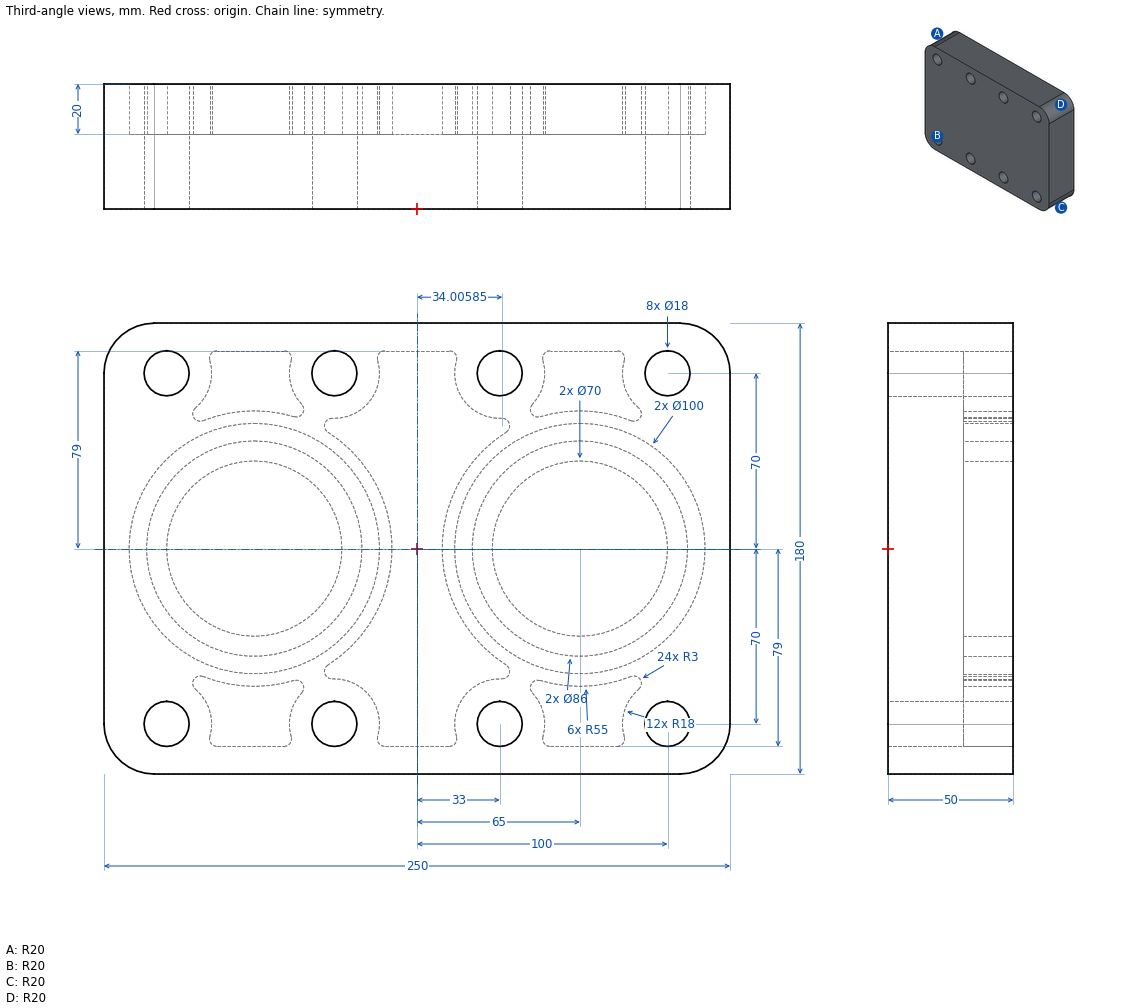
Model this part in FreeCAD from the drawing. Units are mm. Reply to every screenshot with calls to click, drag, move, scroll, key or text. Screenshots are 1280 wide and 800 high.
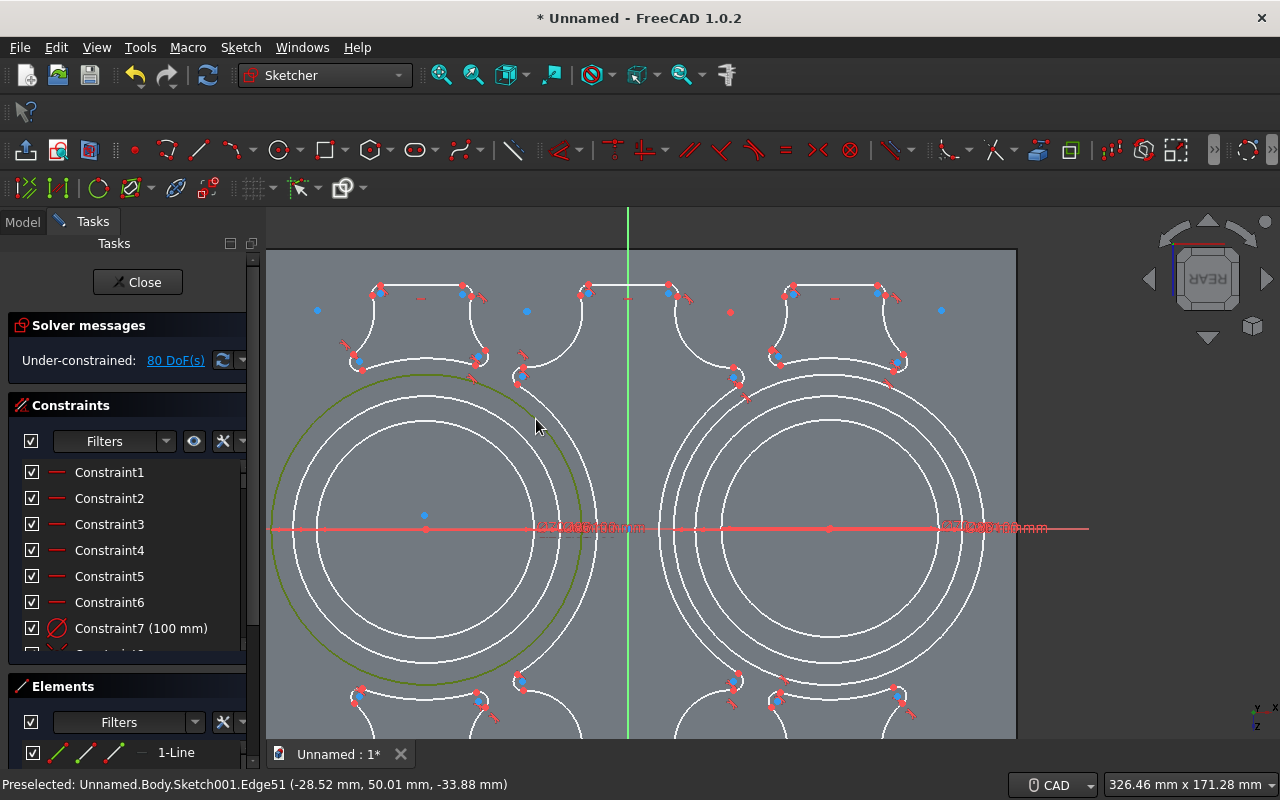
click(583, 596)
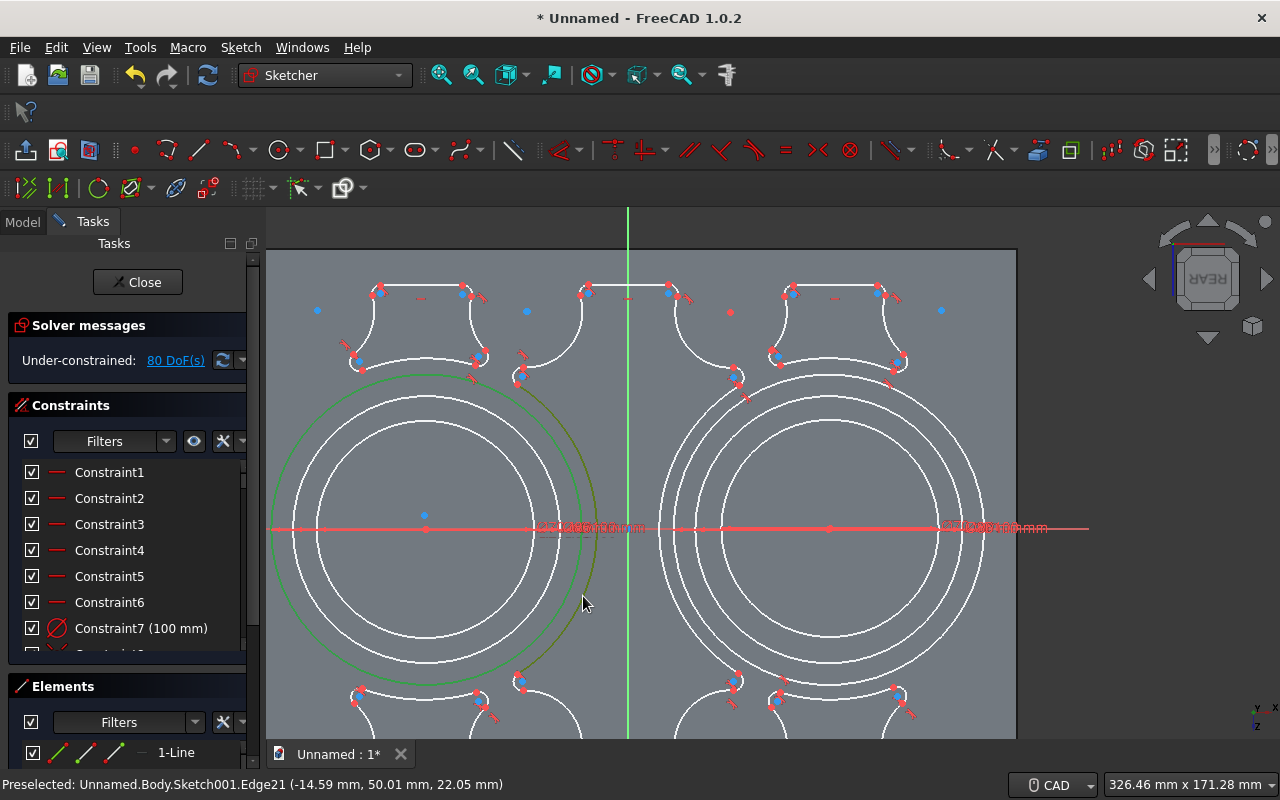
click(614, 150)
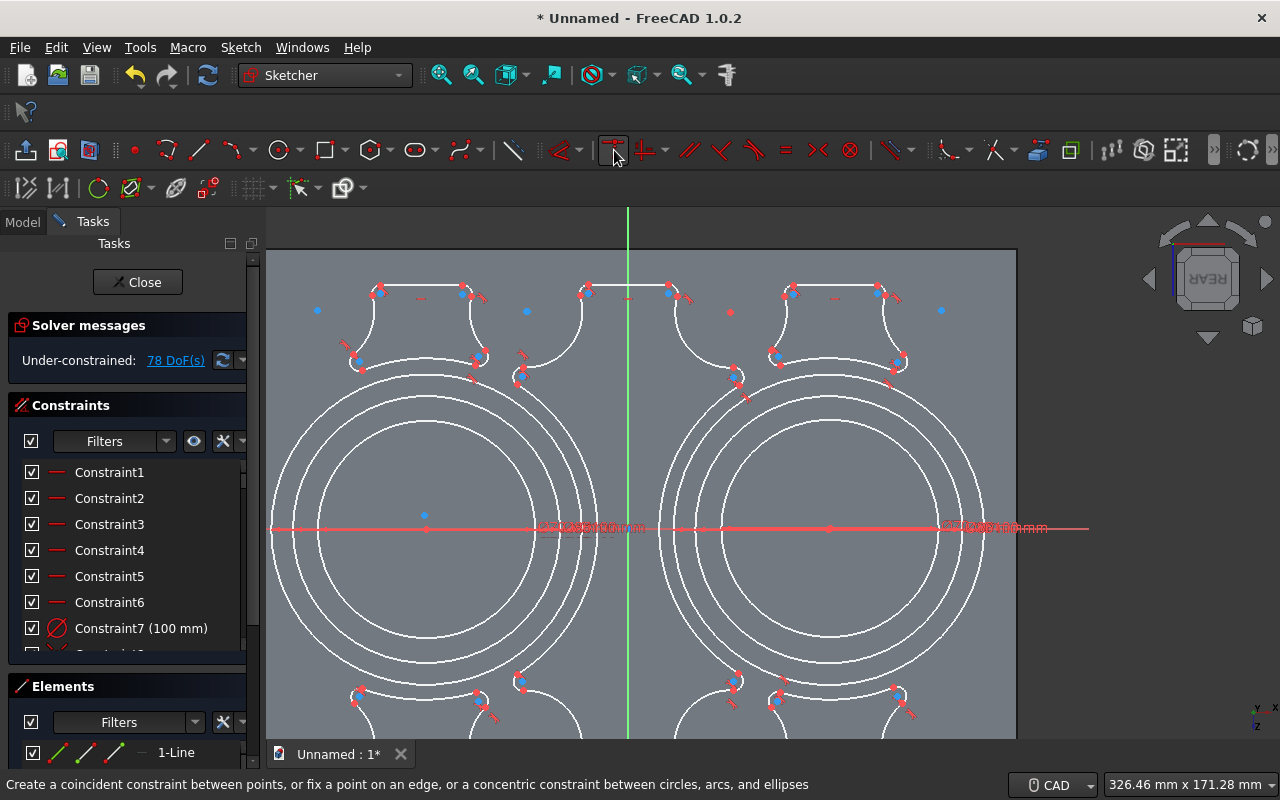
click(554, 360)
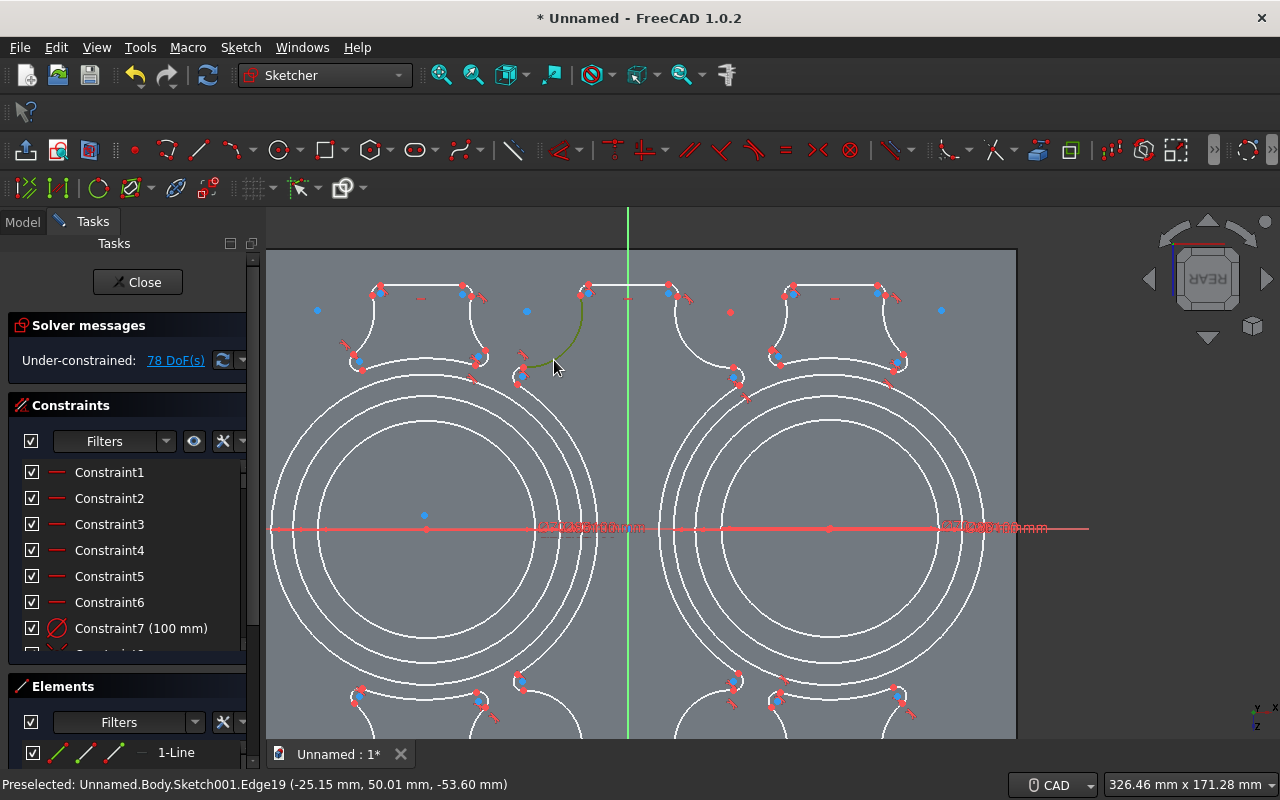
click(470, 314)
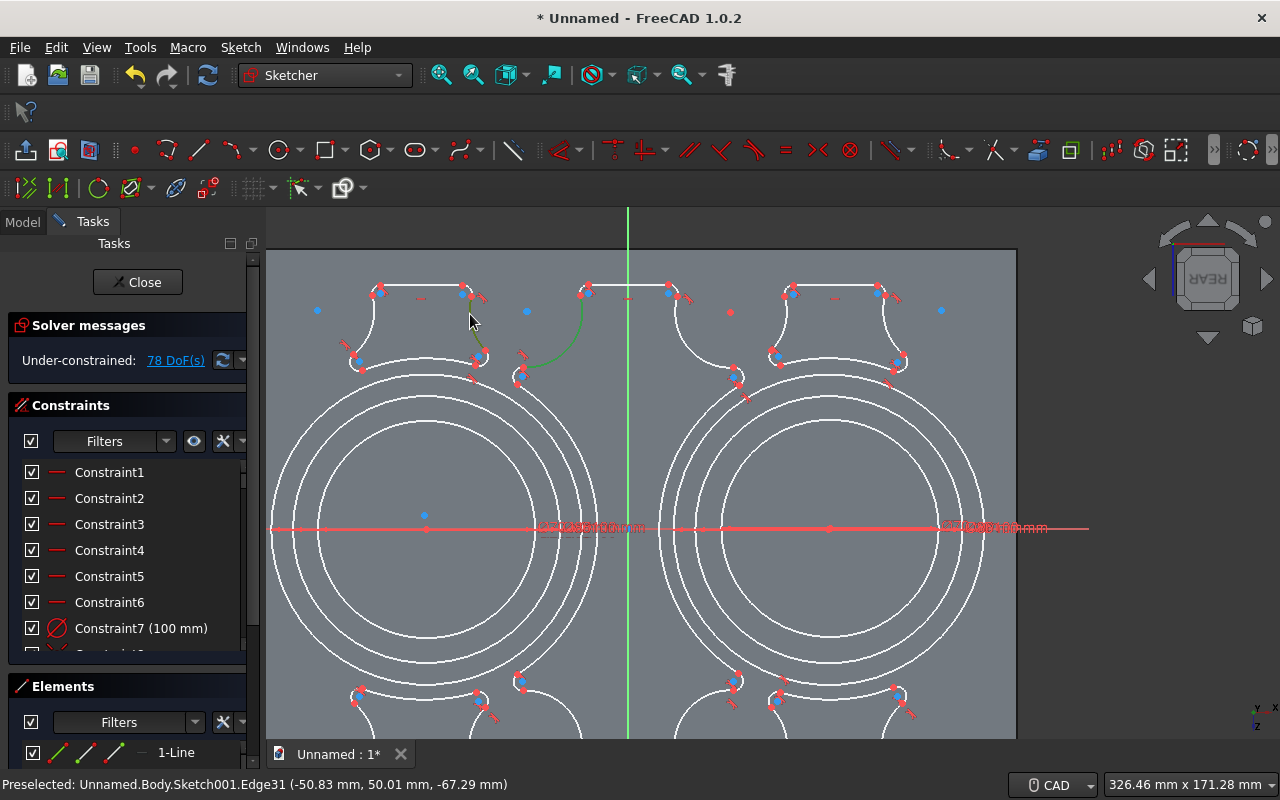
click(614, 150)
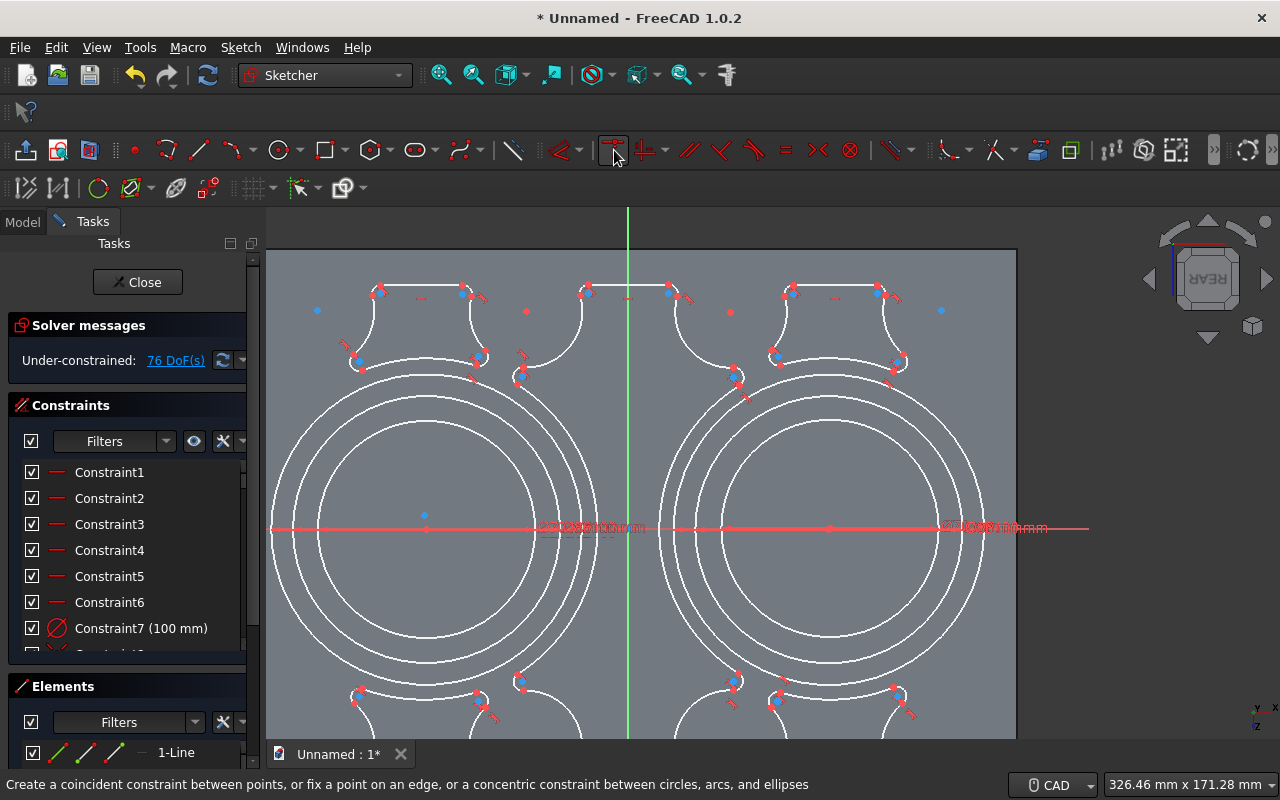
click(554, 698)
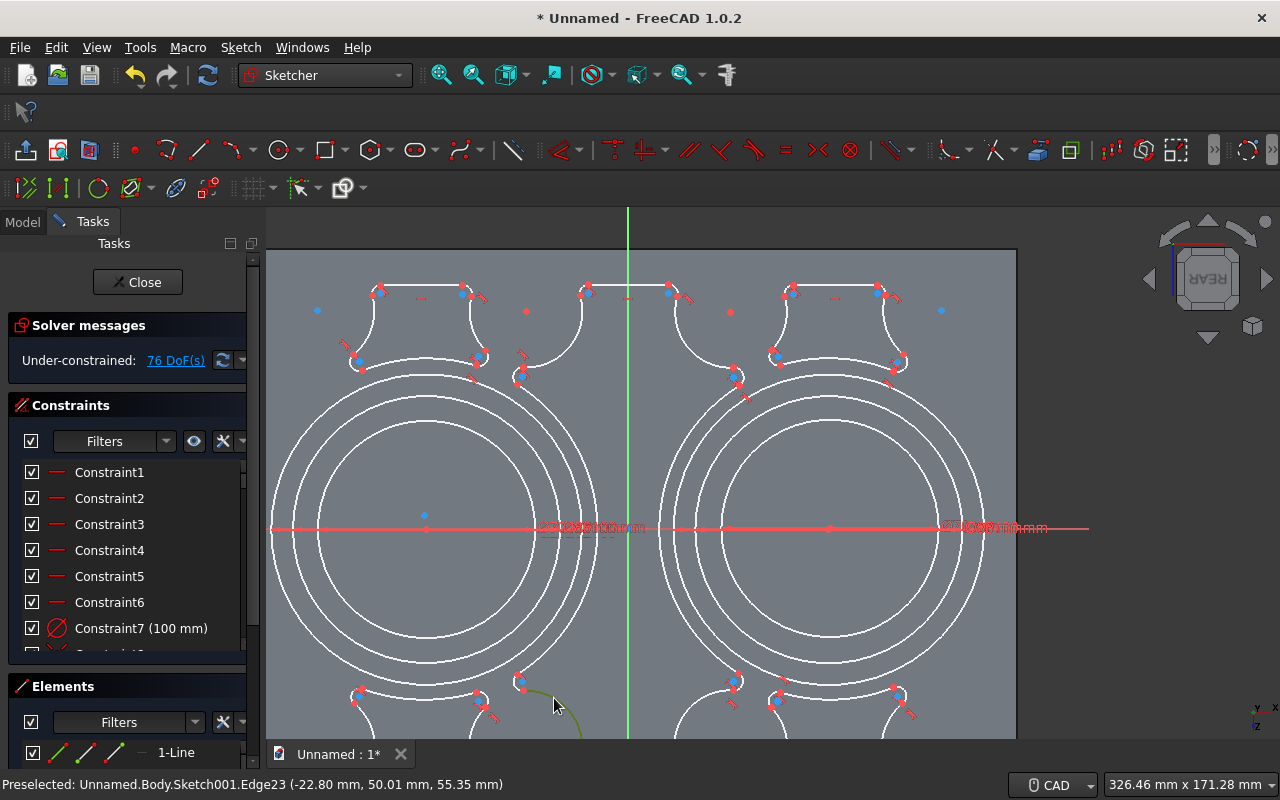
scroll(859, 360, down, 2)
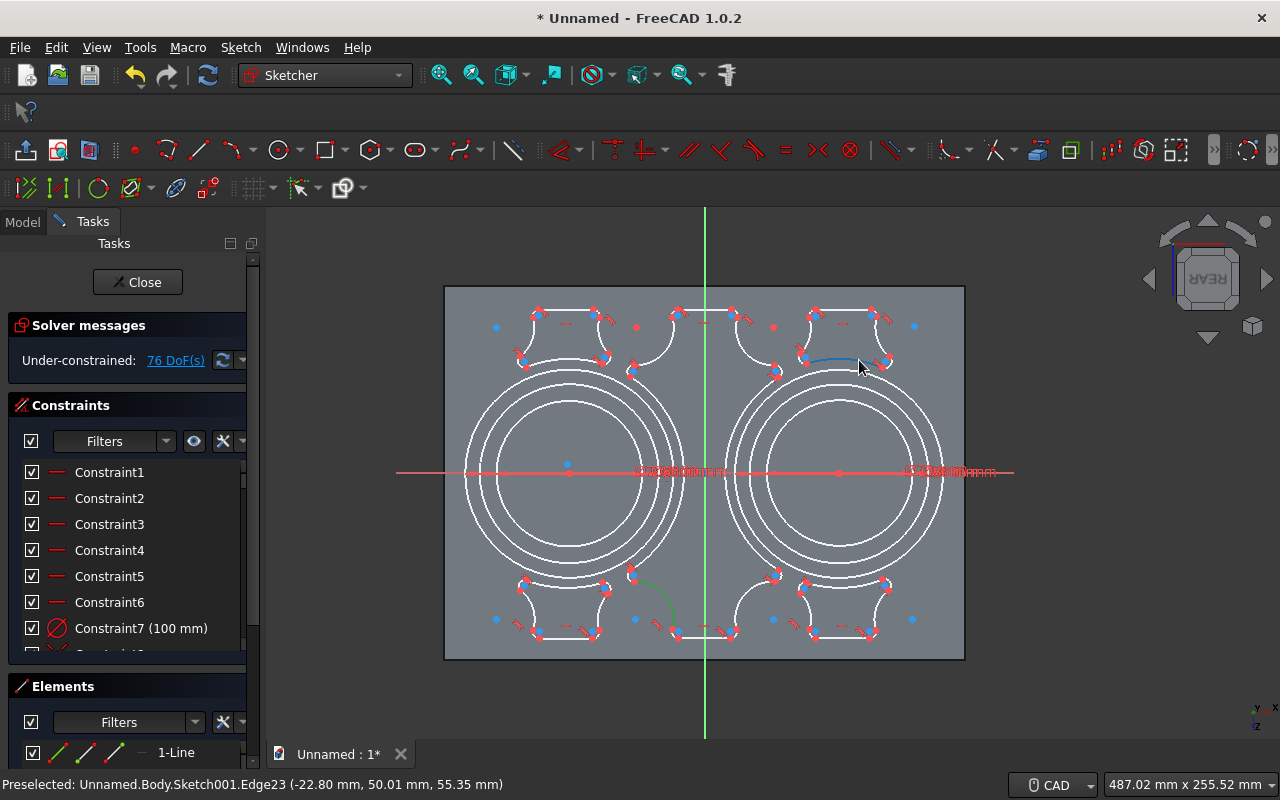
click(602, 603)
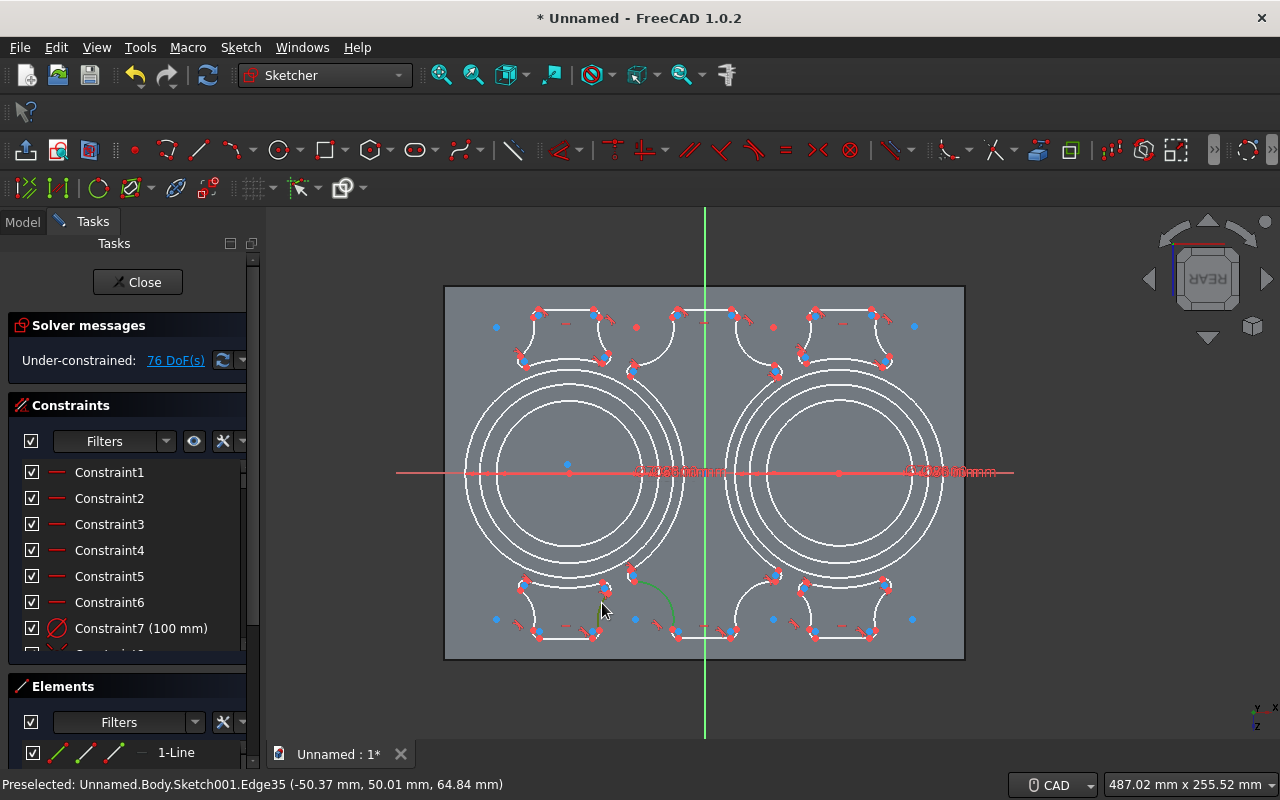
click(614, 150)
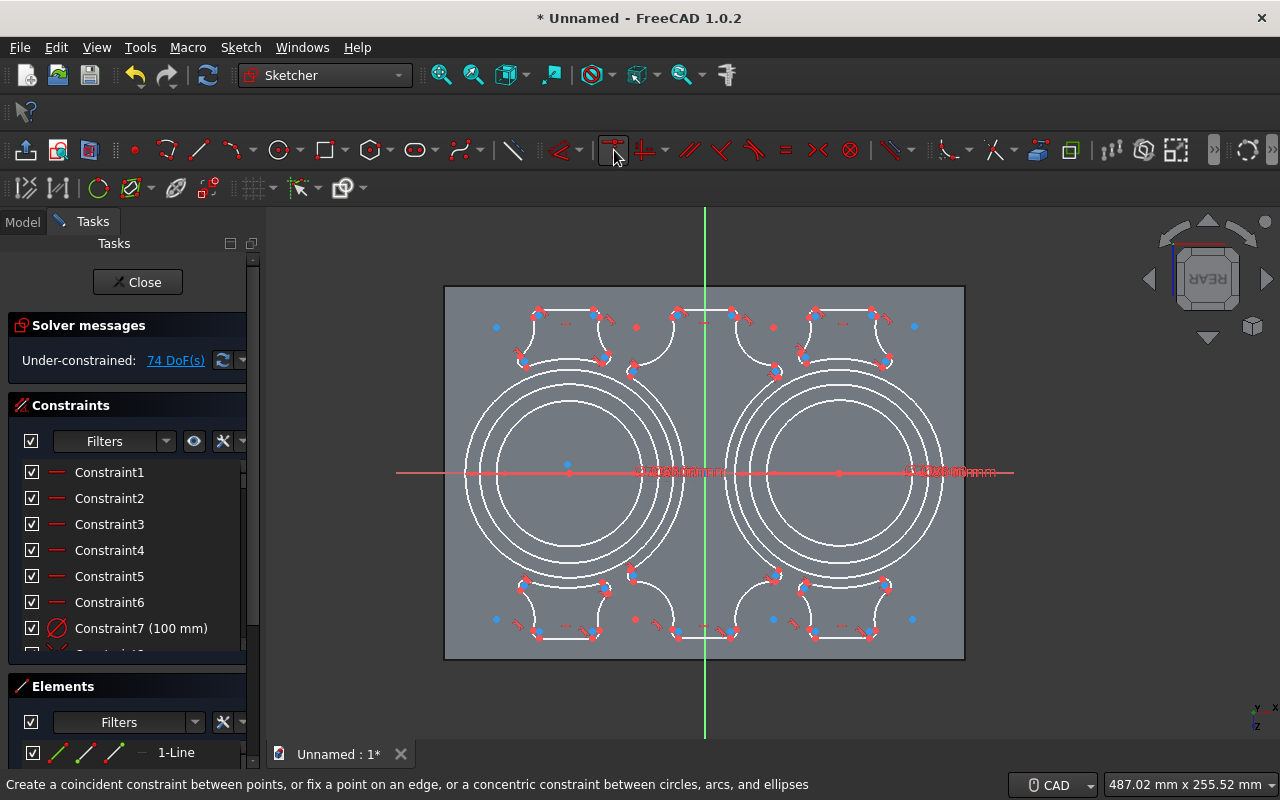
scroll(643, 400, up, 2)